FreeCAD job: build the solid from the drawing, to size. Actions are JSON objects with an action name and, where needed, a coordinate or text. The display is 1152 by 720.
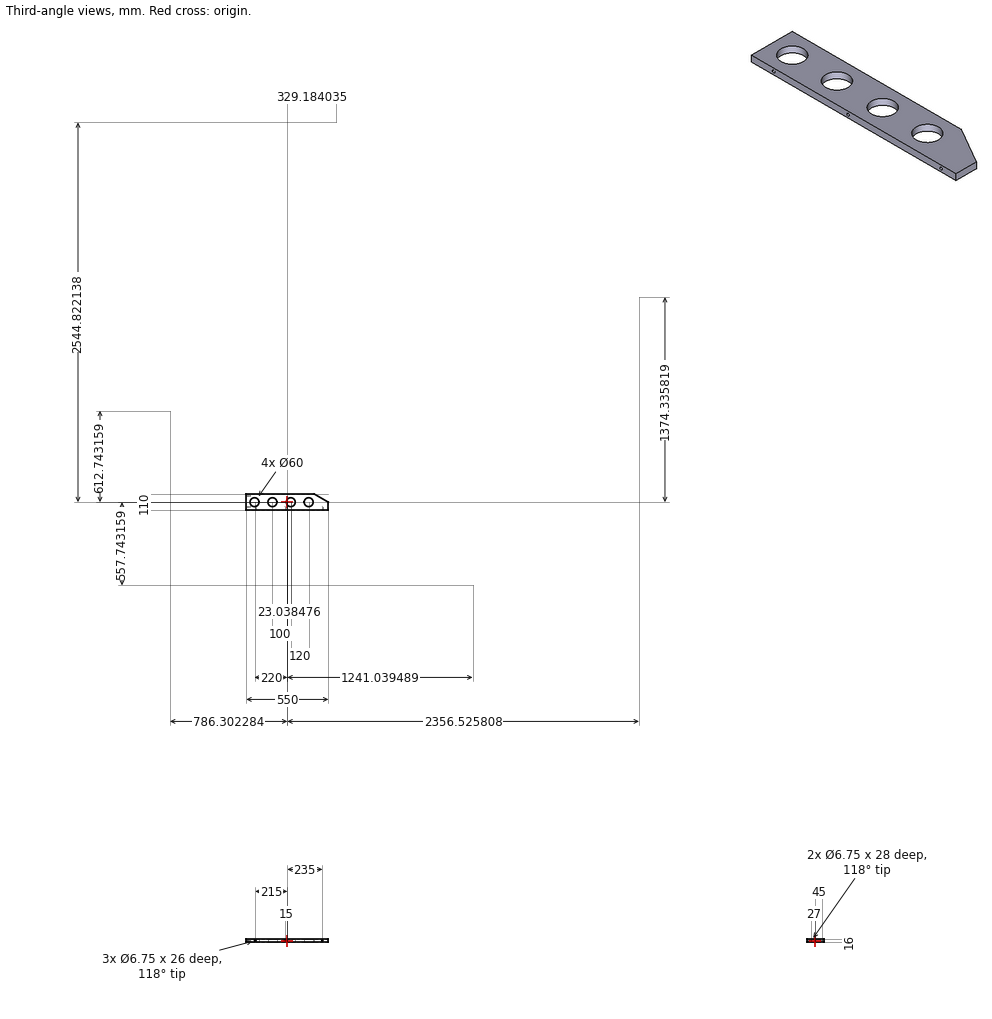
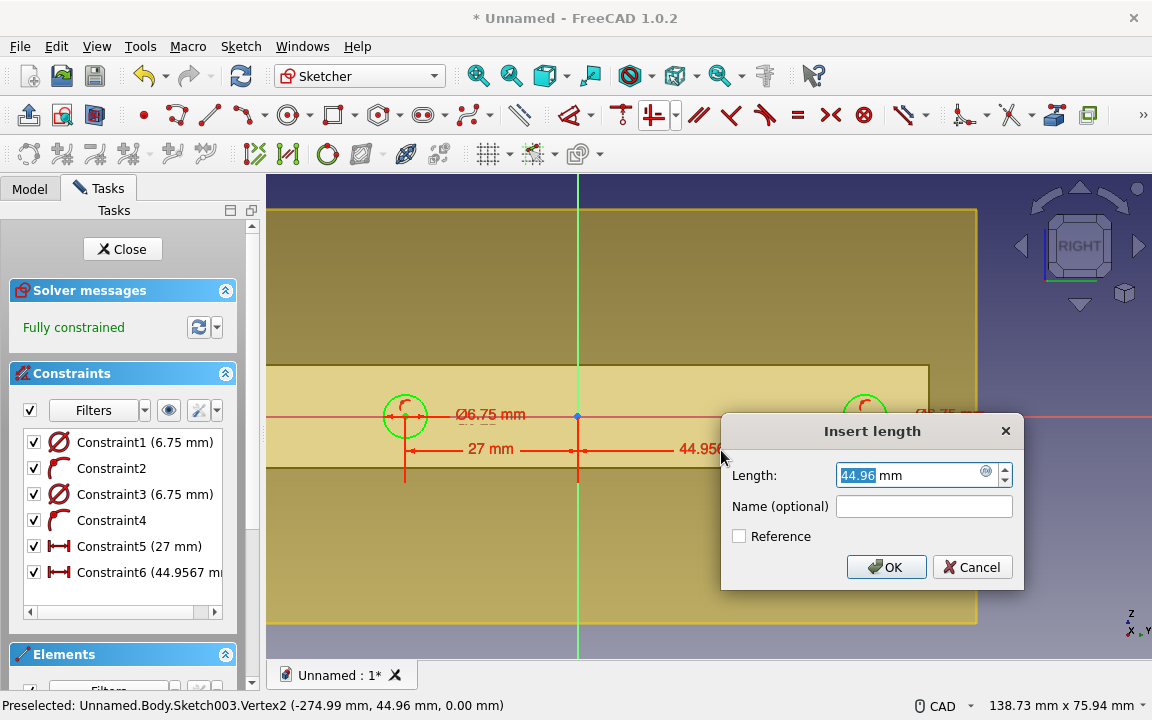
{"action": "type", "text": "45"}
{"action": "key", "text": "Return"}
{"action": "key", "text": "Escape"}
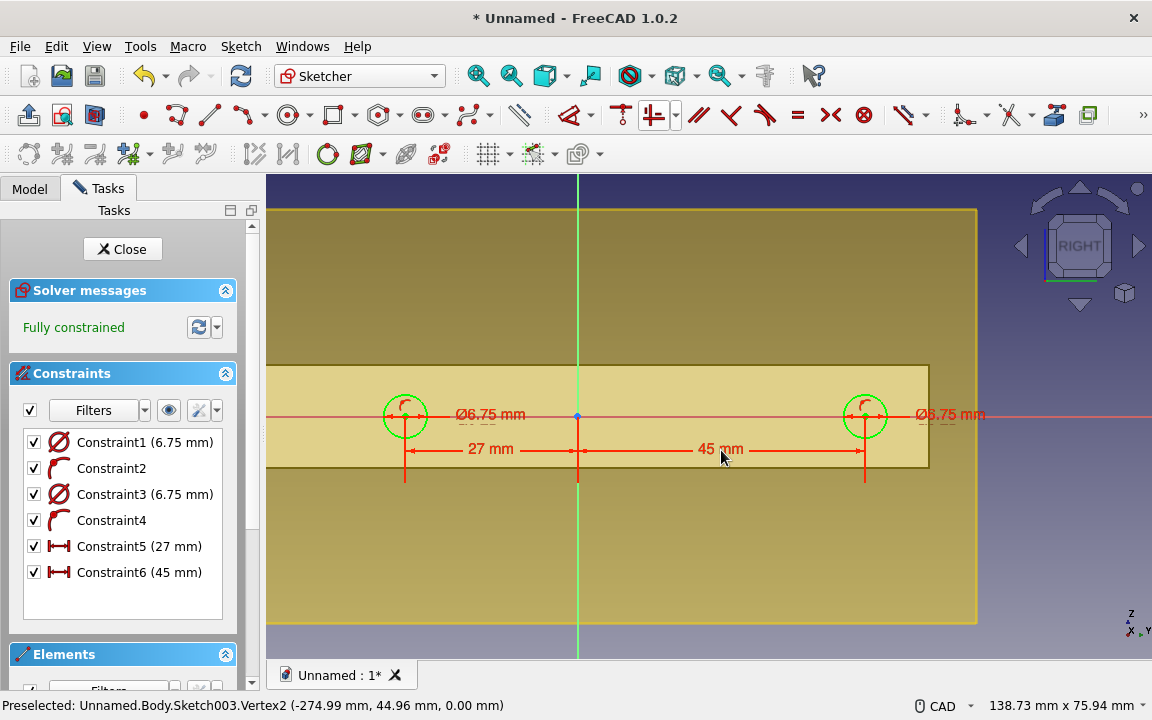
{"action": "left_click", "coordinate": [123, 249]}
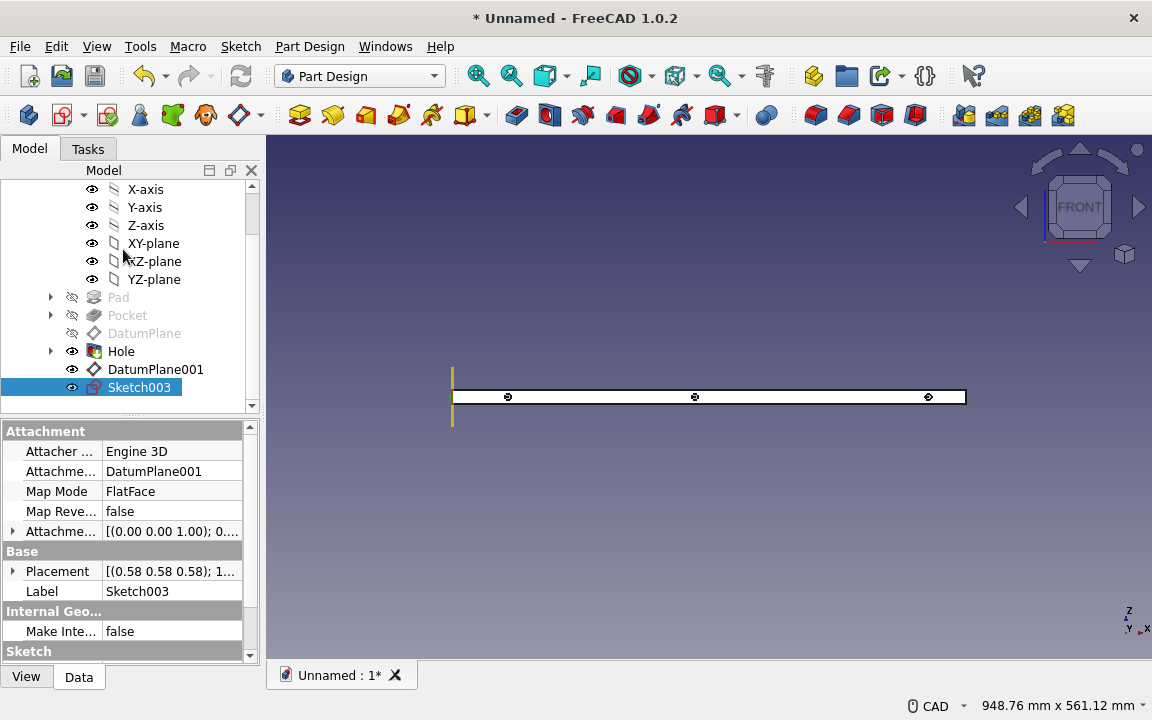
{"action": "left_click", "coordinate": [550, 116]}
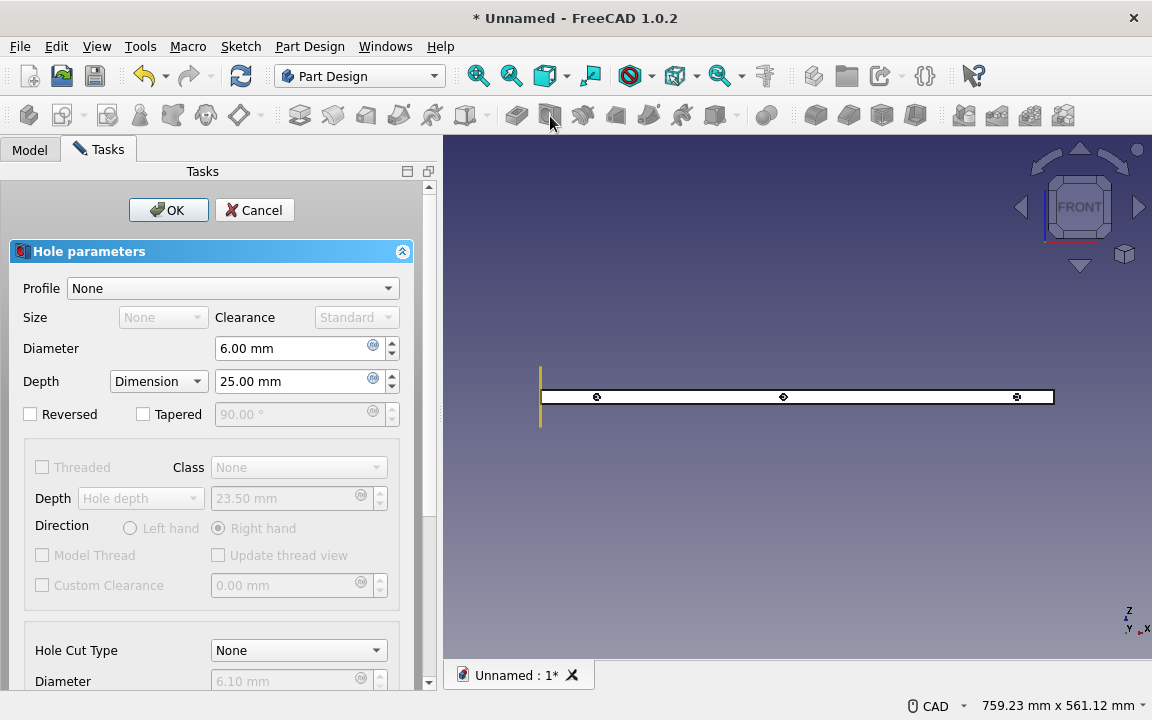
{"action": "triple_click", "coordinate": [300, 348]}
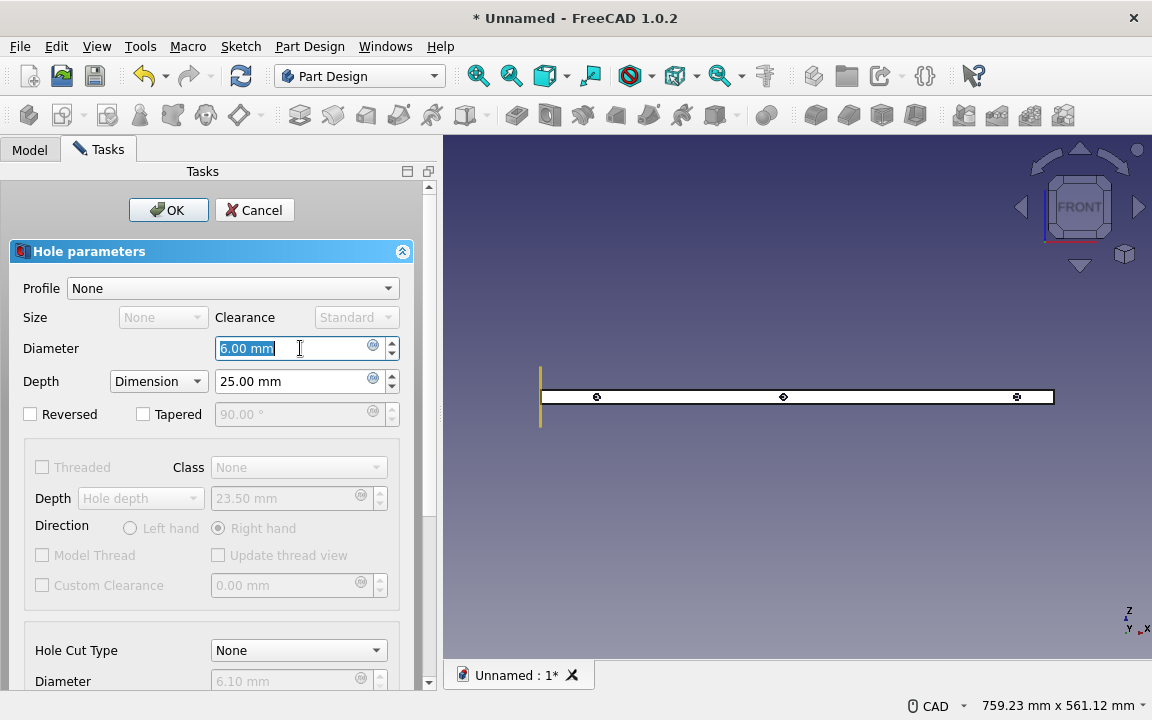
{"action": "type", "text": "6.75"}
{"action": "key", "text": "Tab"}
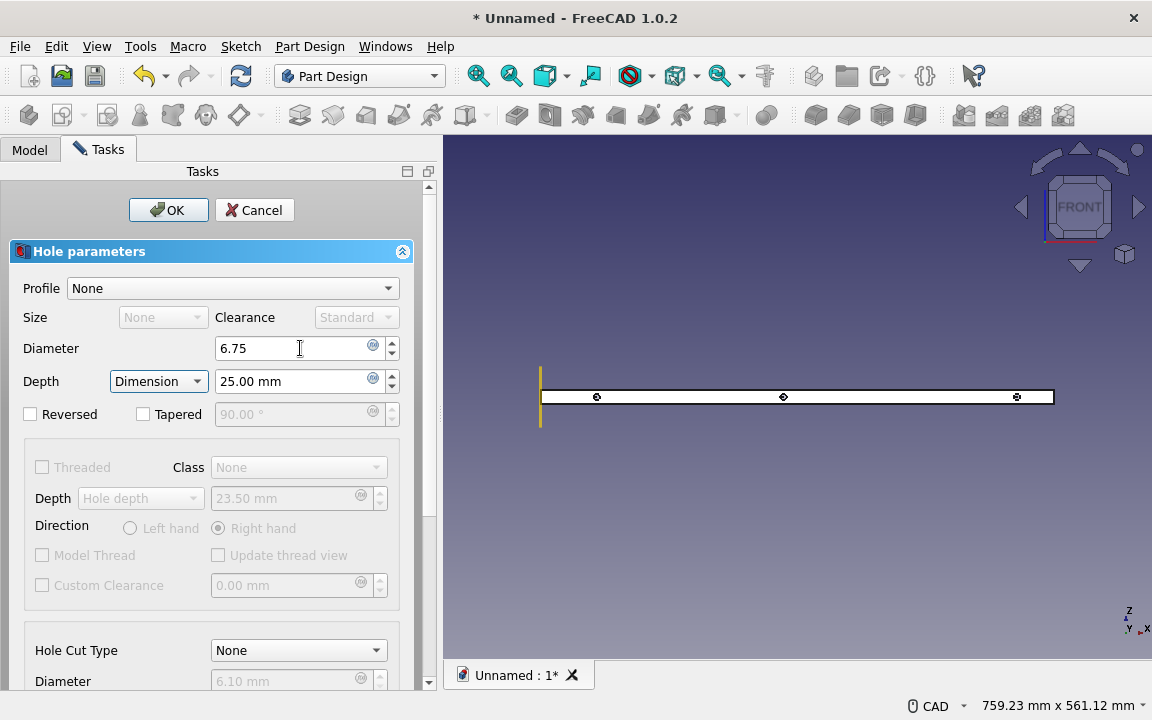
{"action": "triple_click", "coordinate": [300, 382]}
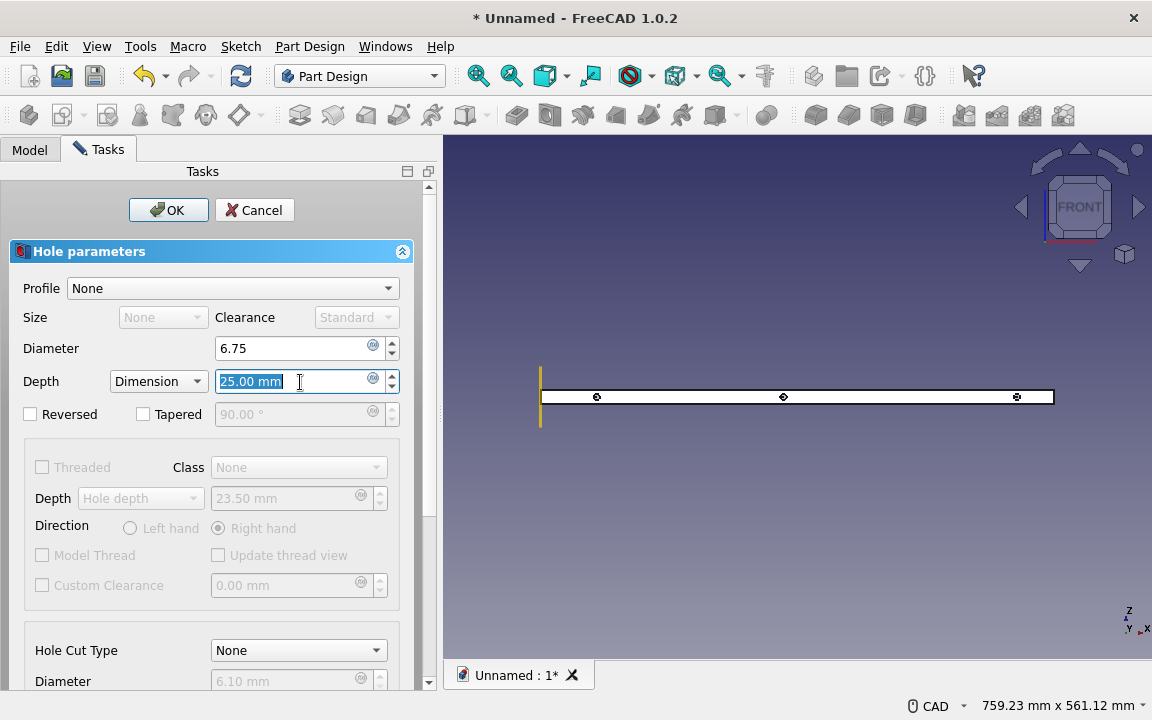
{"action": "type", "text": "28"}
{"action": "key", "text": "Tab"}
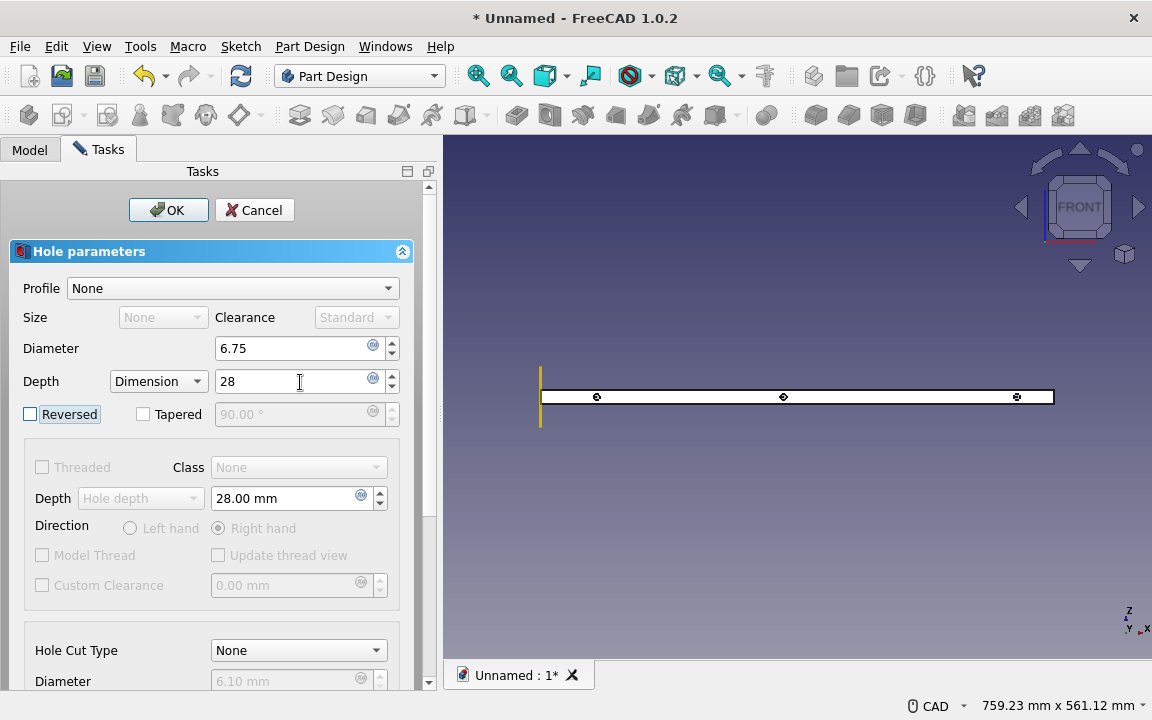
{"action": "left_click", "coordinate": [31, 414]}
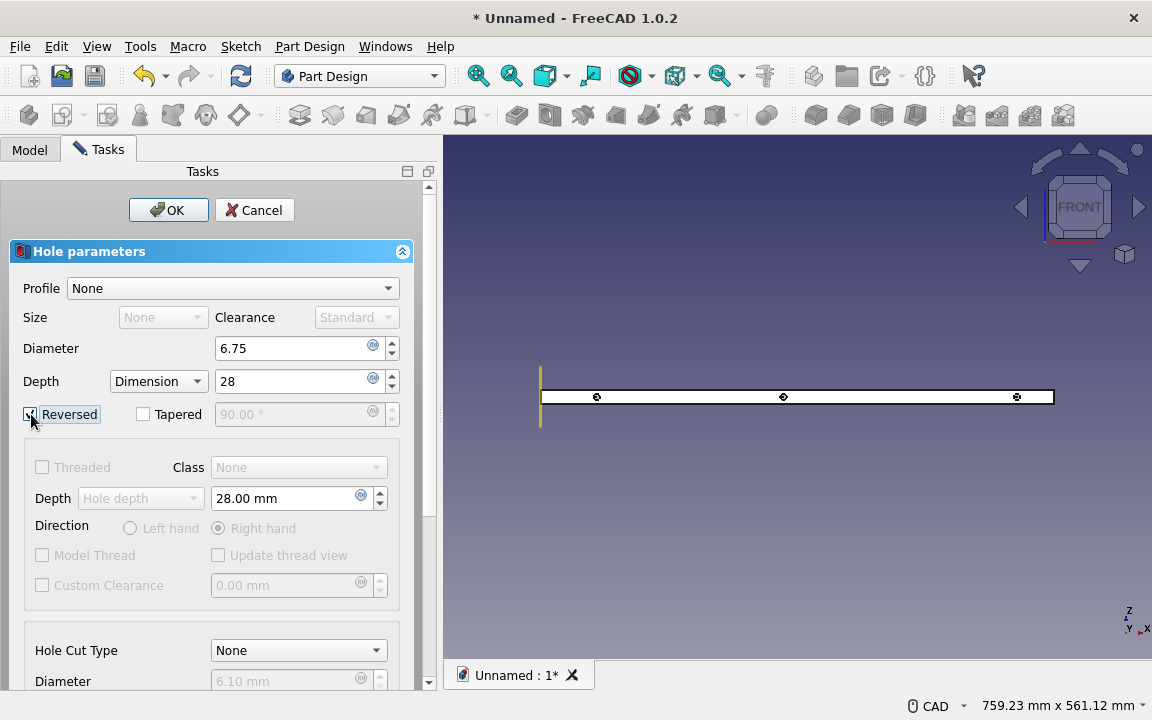
{"action": "left_click", "coordinate": [169, 210]}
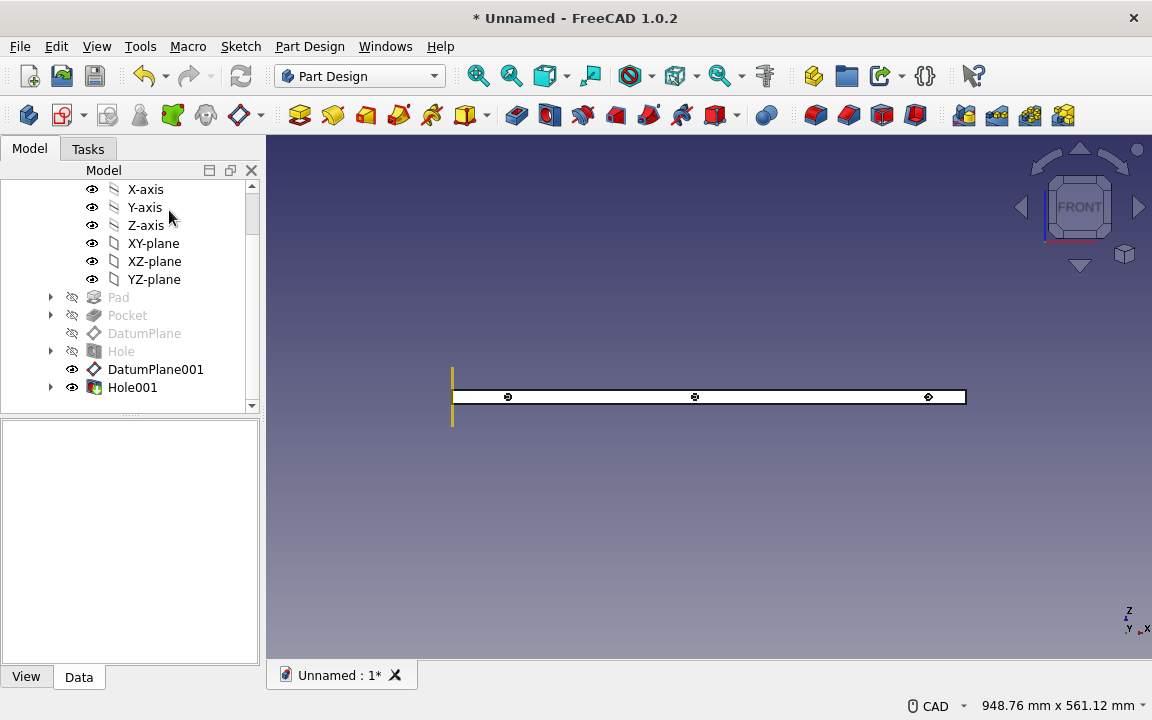
{"action": "left_click", "coordinate": [117, 369]}
{"action": "key", "text": "space"}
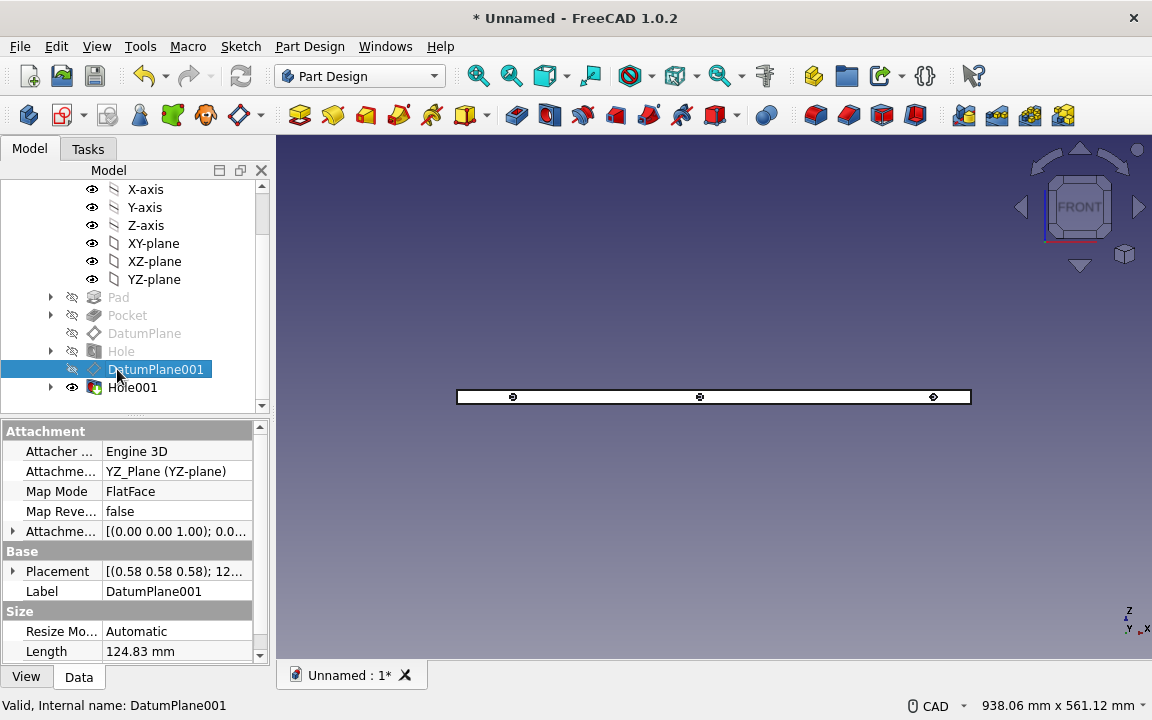
{"action": "key", "text": "0"}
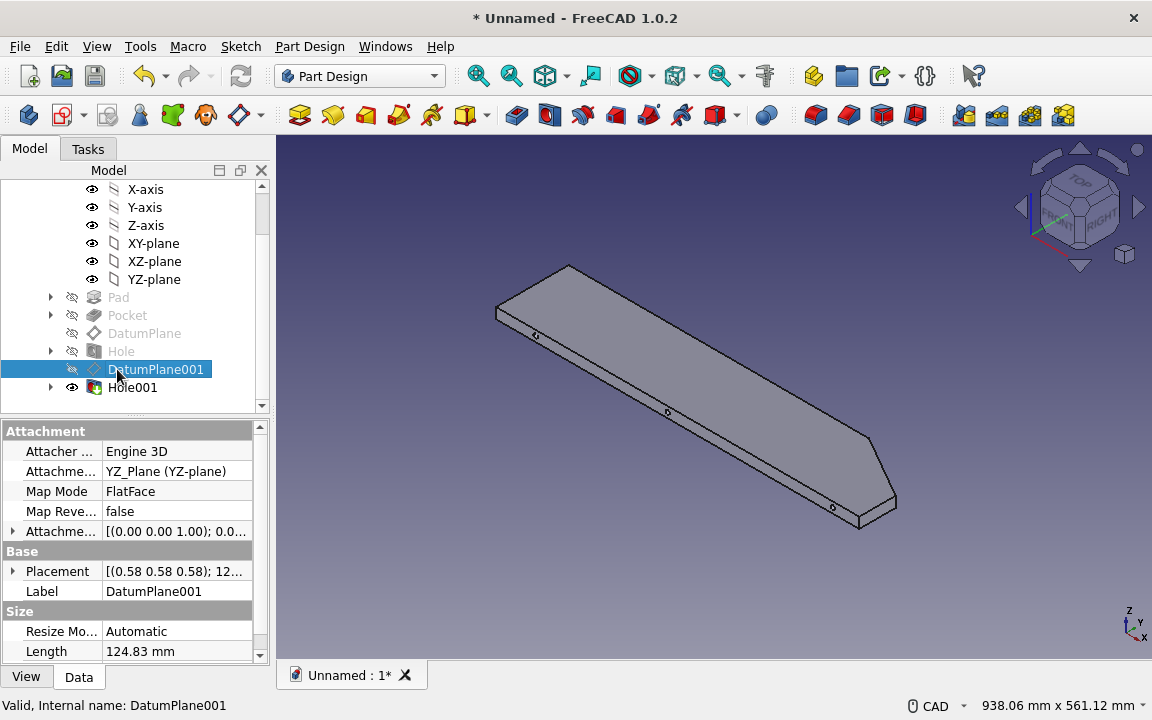
{"action": "left_click", "coordinate": [818, 450]}